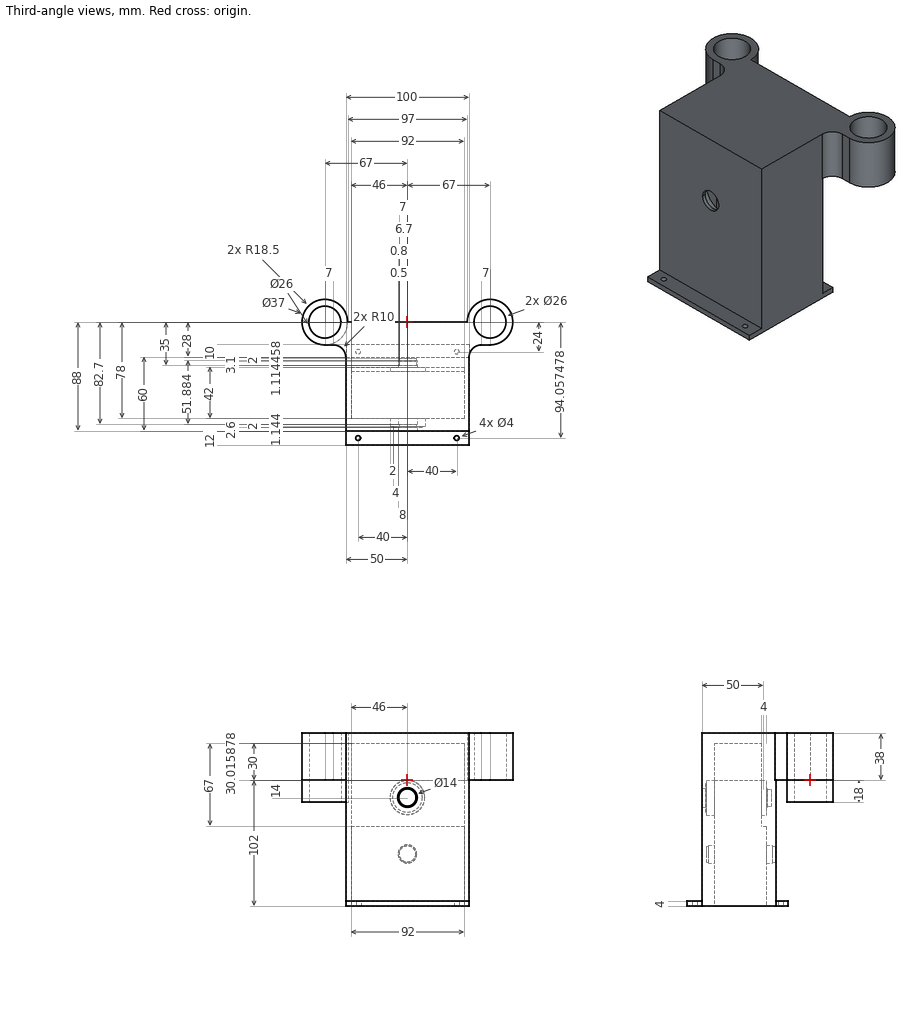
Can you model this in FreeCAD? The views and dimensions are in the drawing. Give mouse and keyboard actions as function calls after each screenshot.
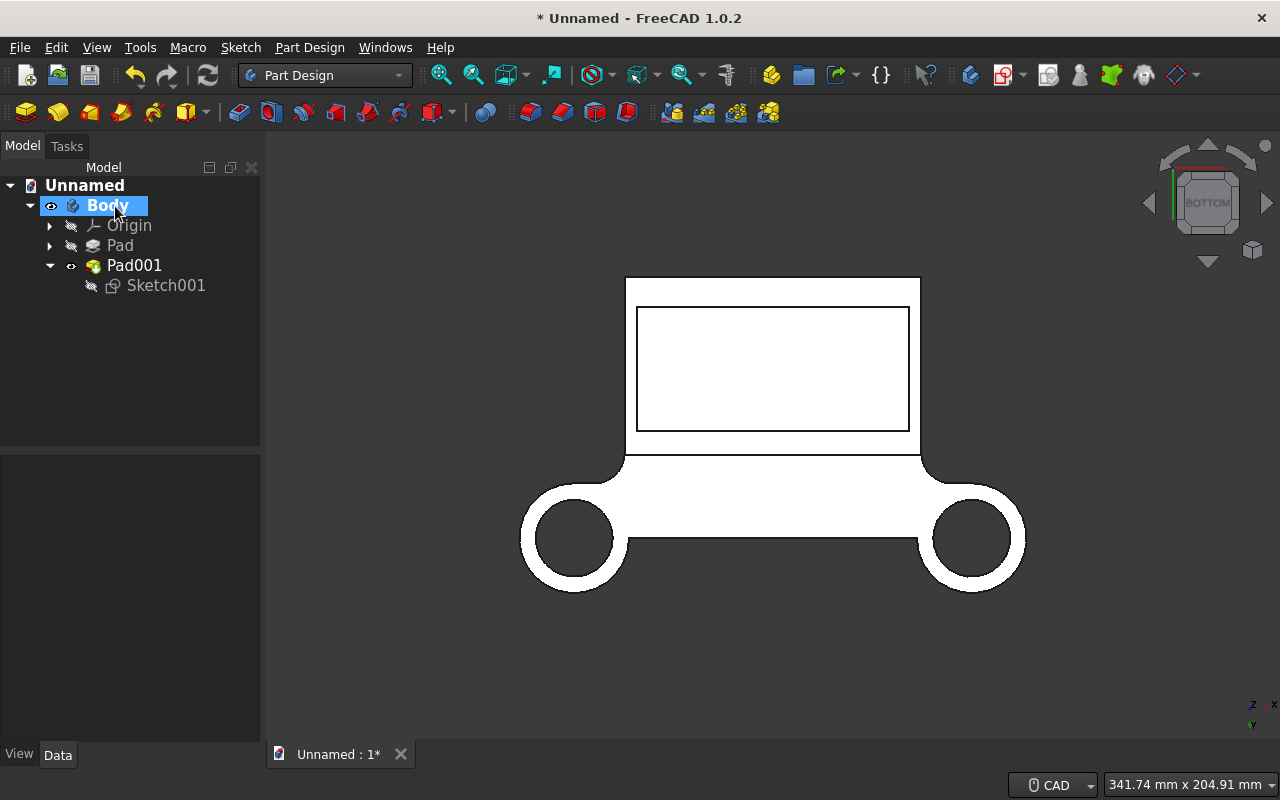
key(0)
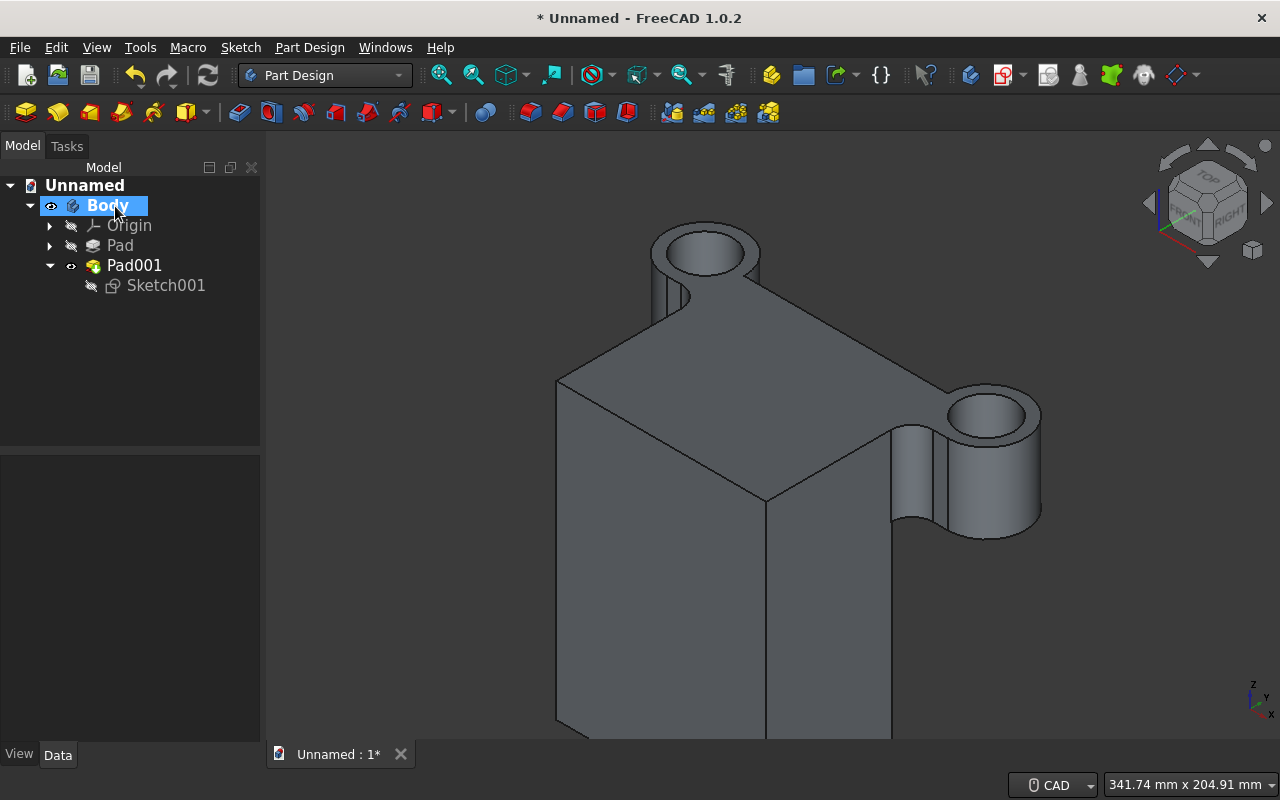
key(v)
key(f)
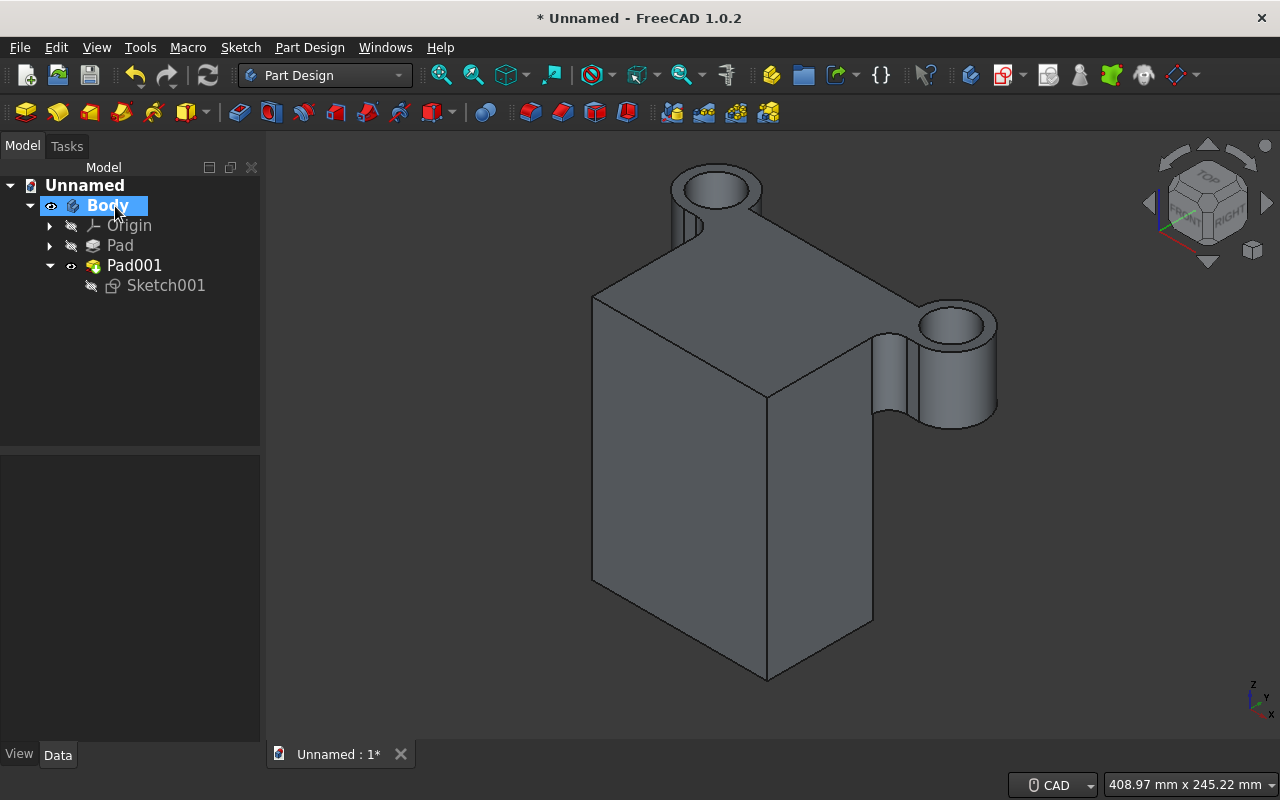
click(680, 447)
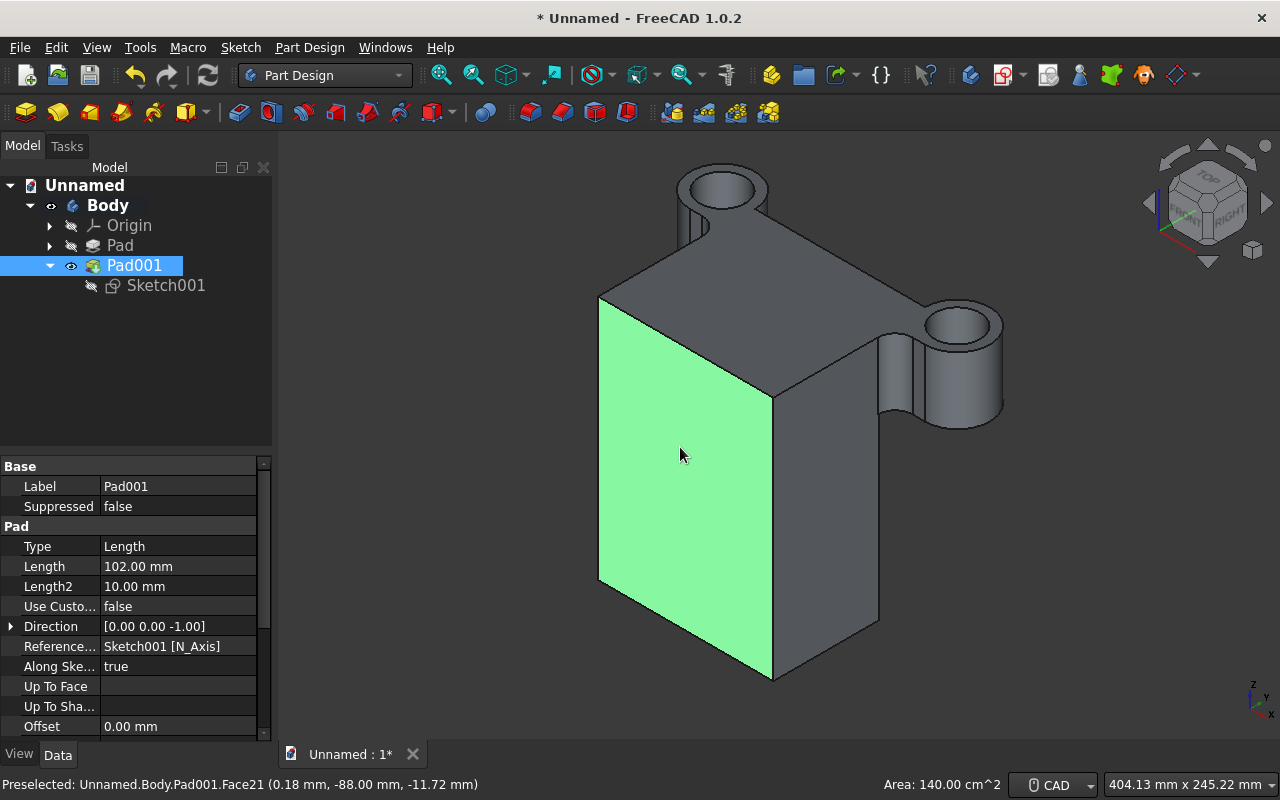
click(1004, 76)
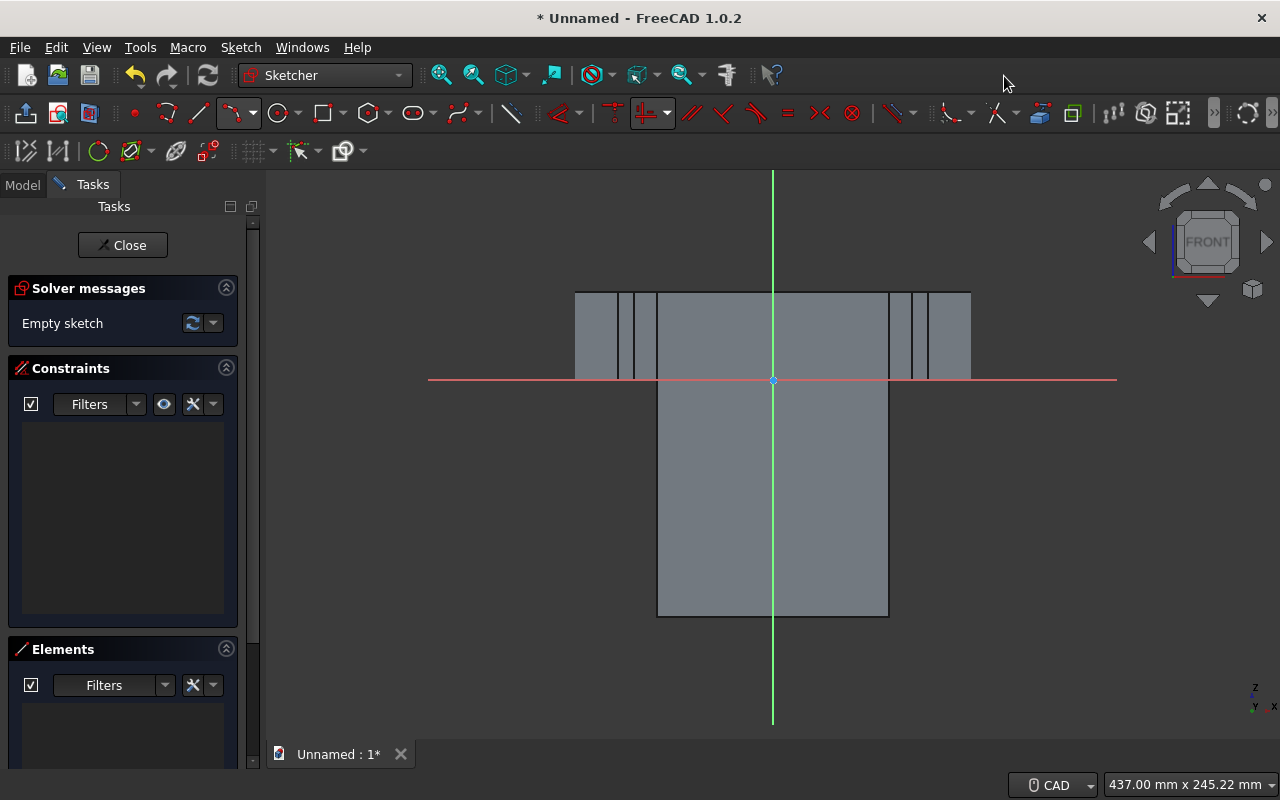
scroll(784, 397, up, 10)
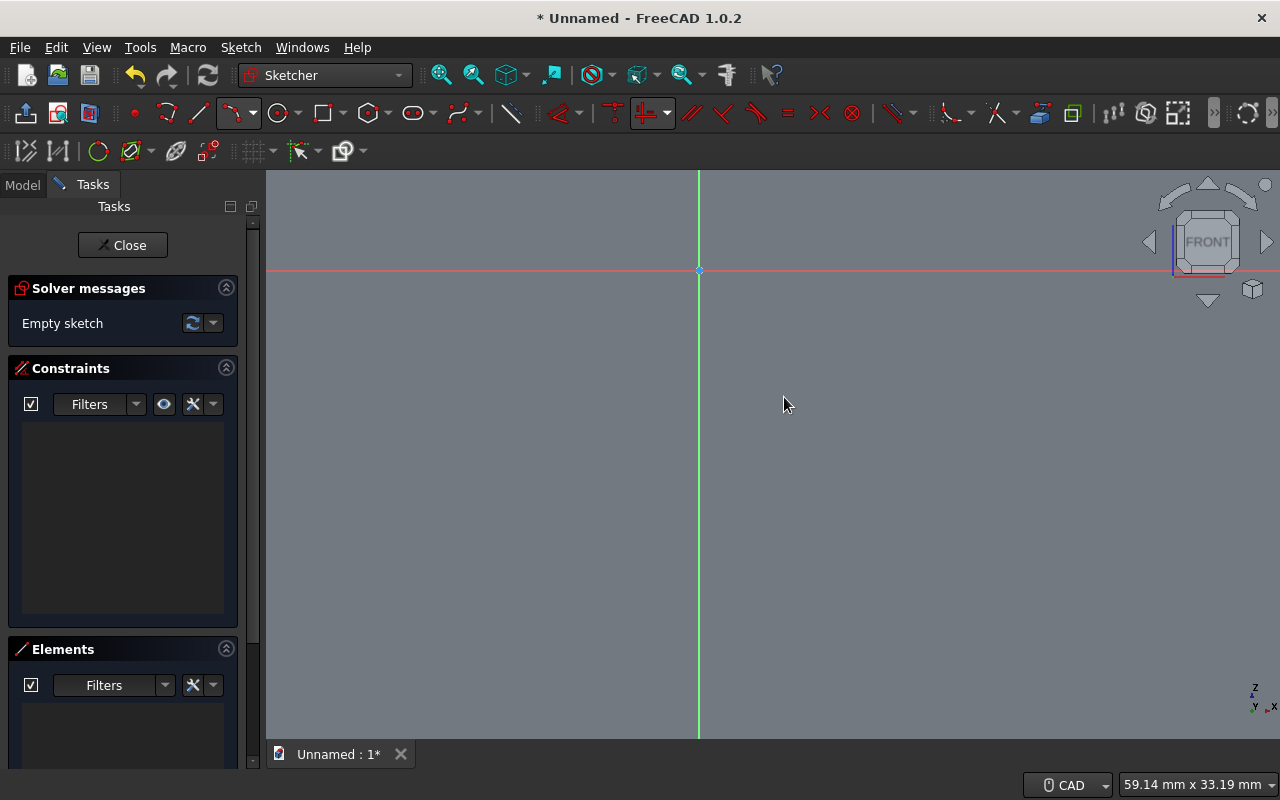
click(278, 114)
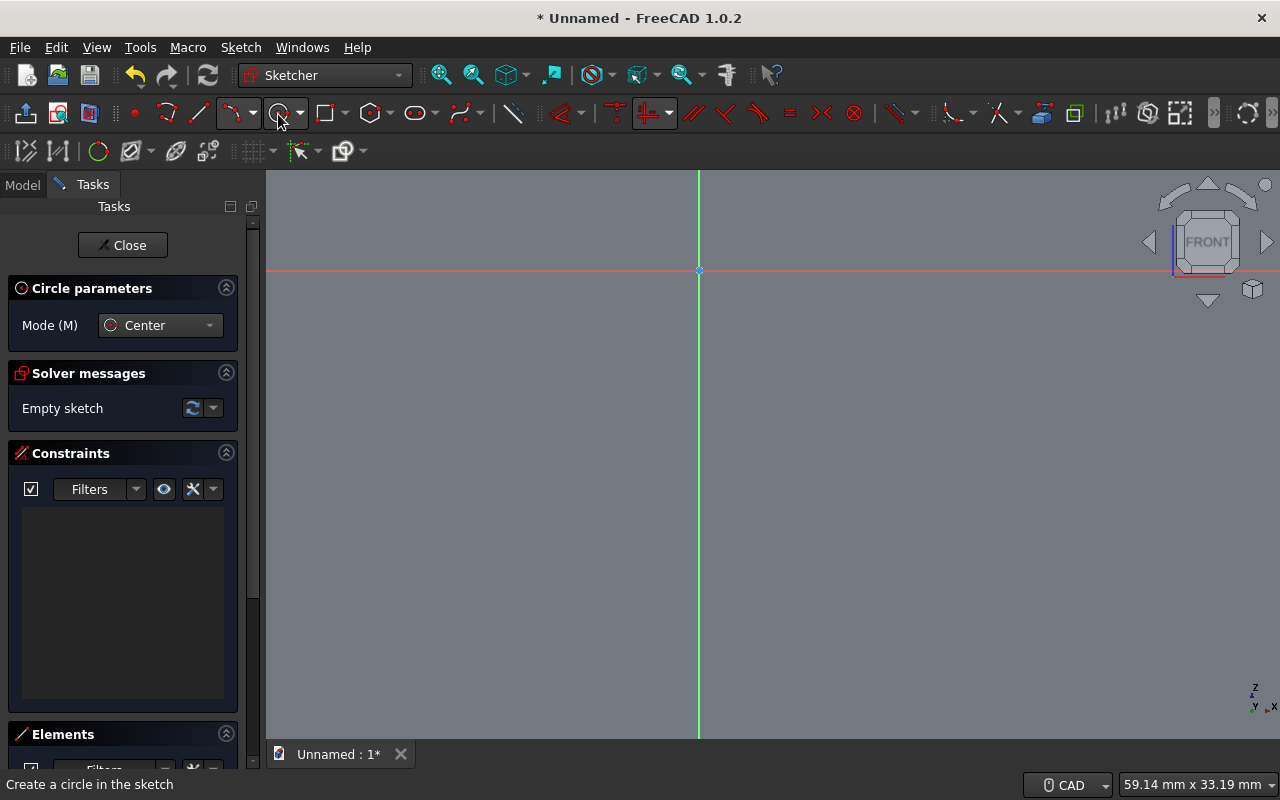
click(699, 511)
click(784, 426)
key(Escape)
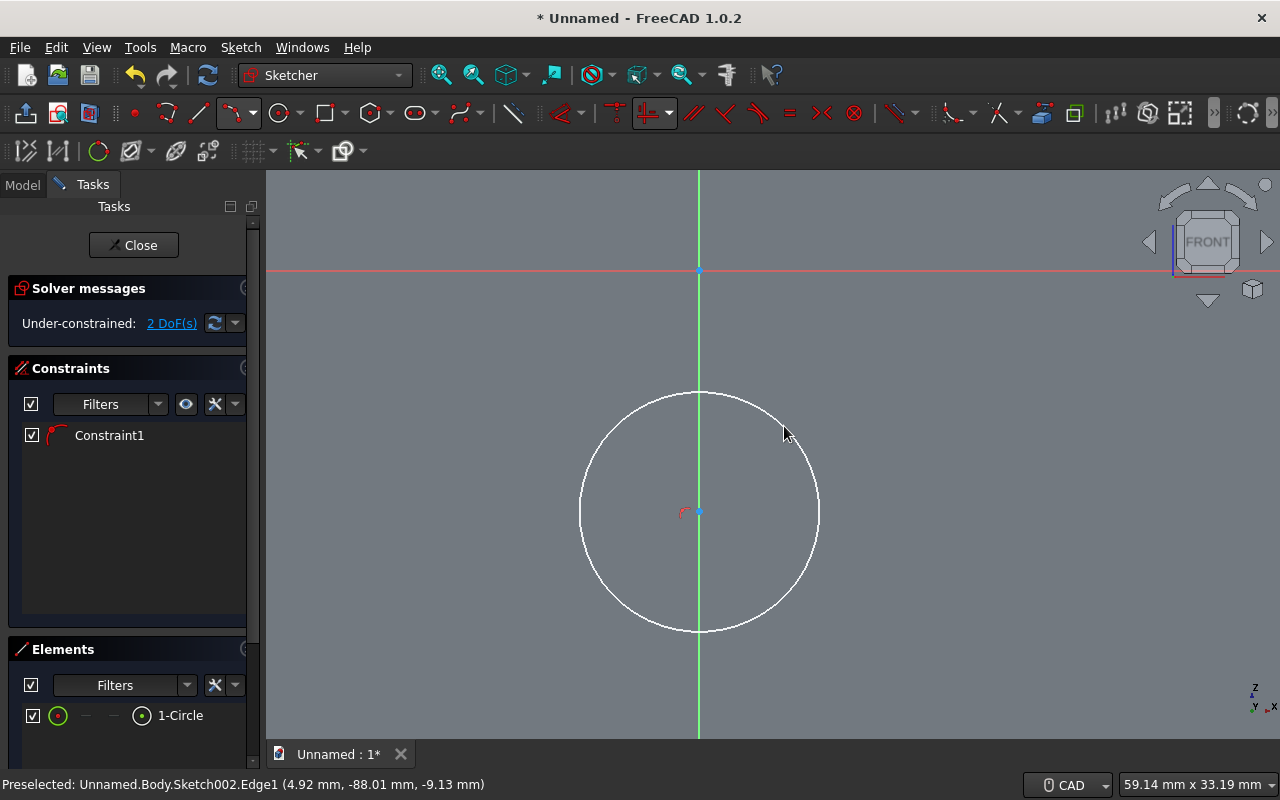
key(d)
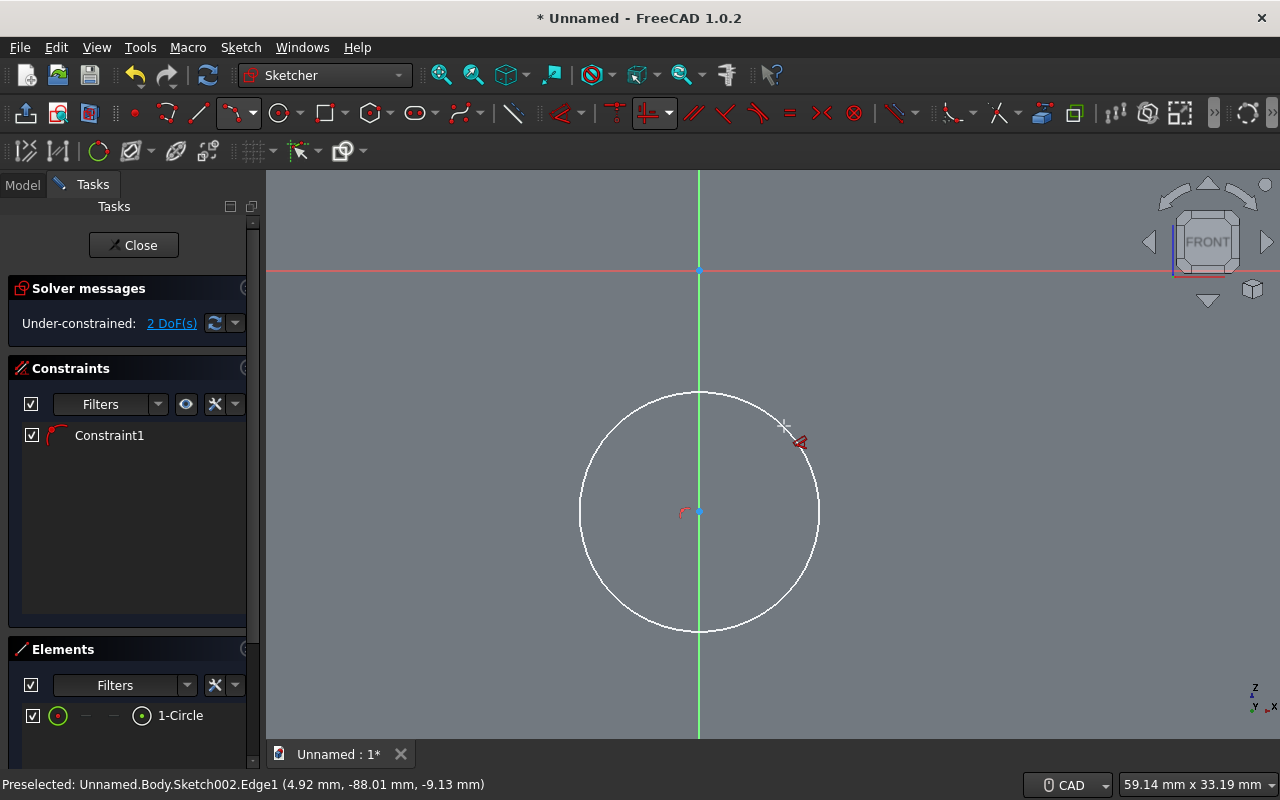
click(784, 427)
click(807, 404)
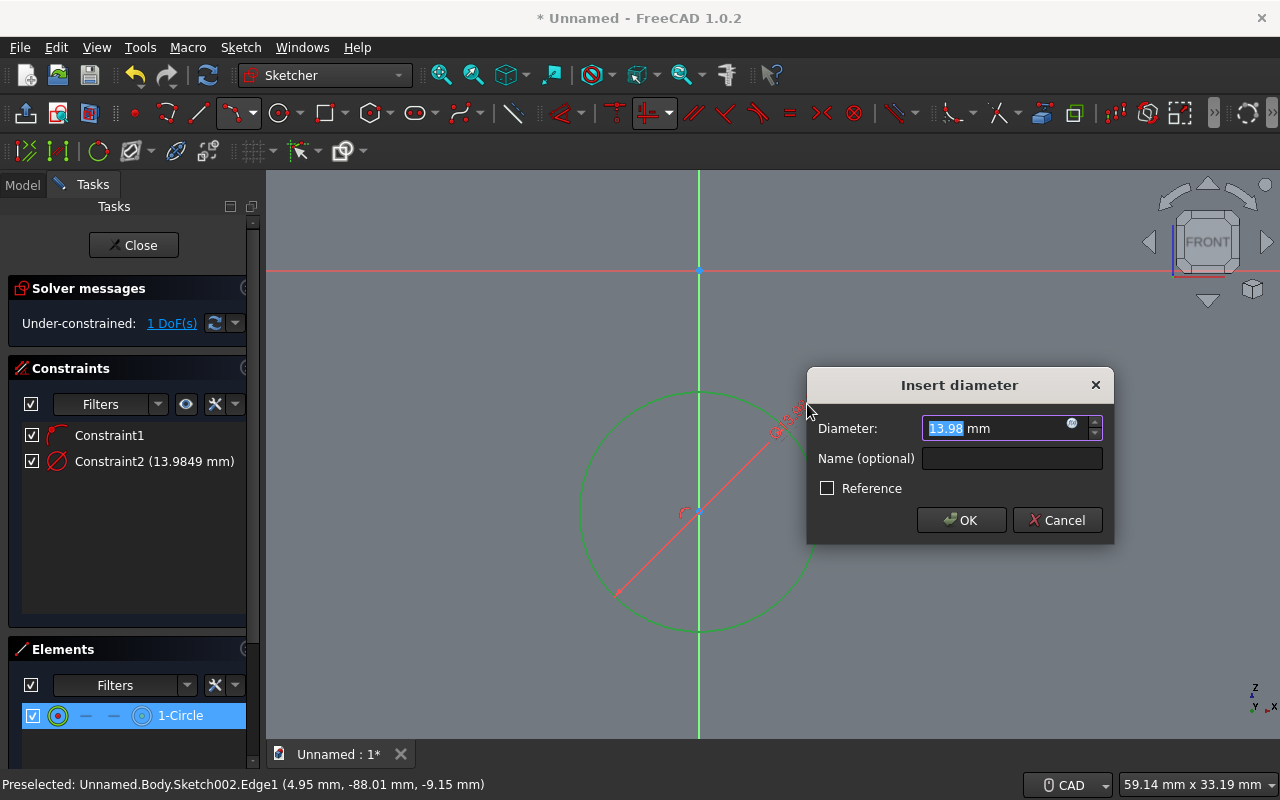
text(14)
key(Return)